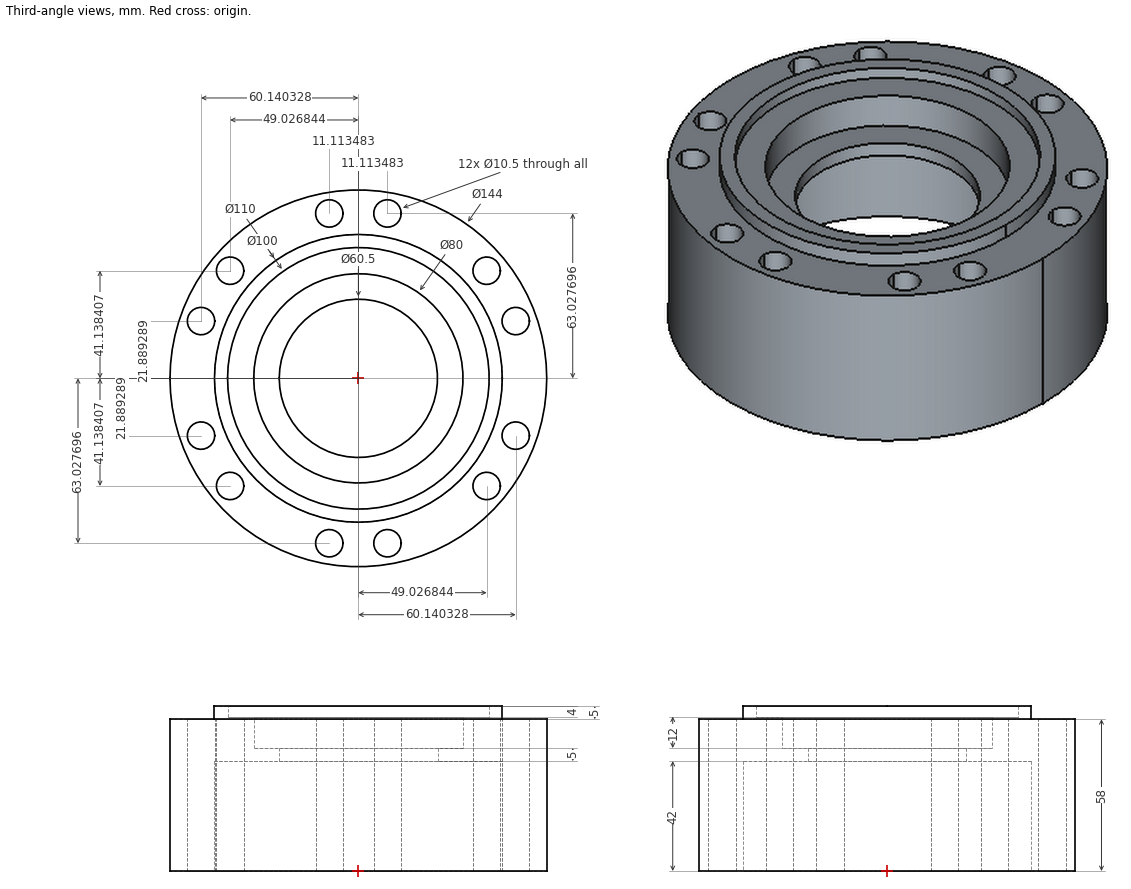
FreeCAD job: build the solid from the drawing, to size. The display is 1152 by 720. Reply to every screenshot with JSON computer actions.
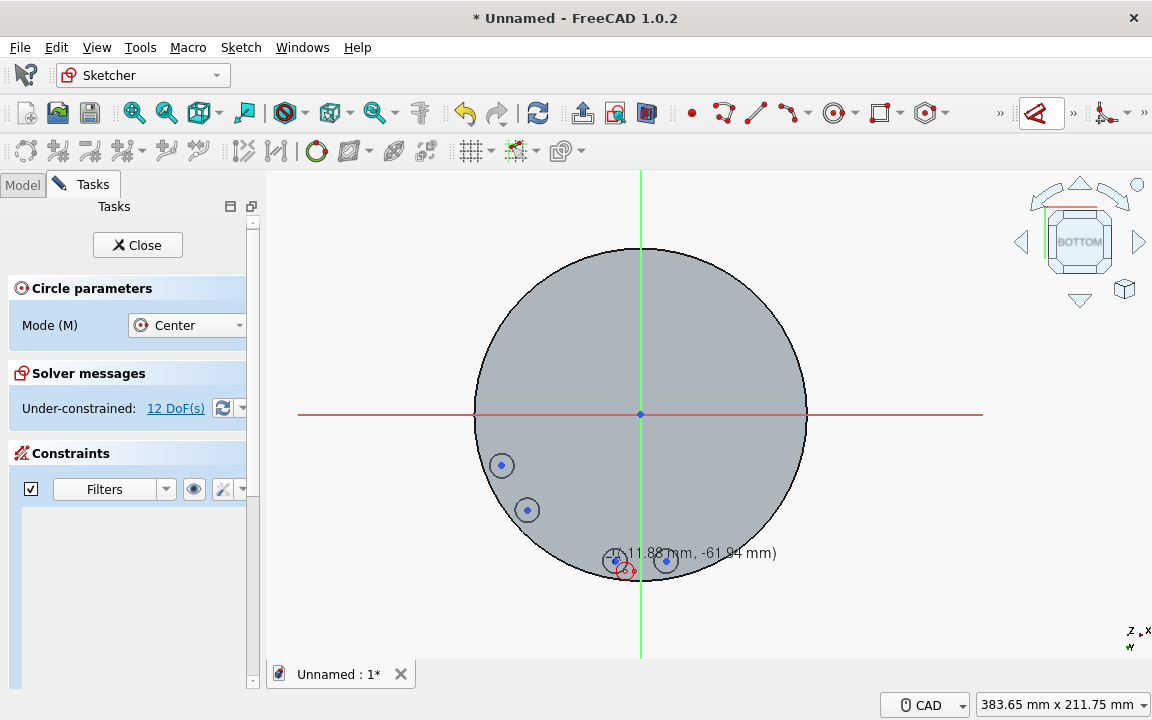
{"action": "scroll", "coordinate": [502, 364], "scroll_direction": "up", "scroll_amount": 4}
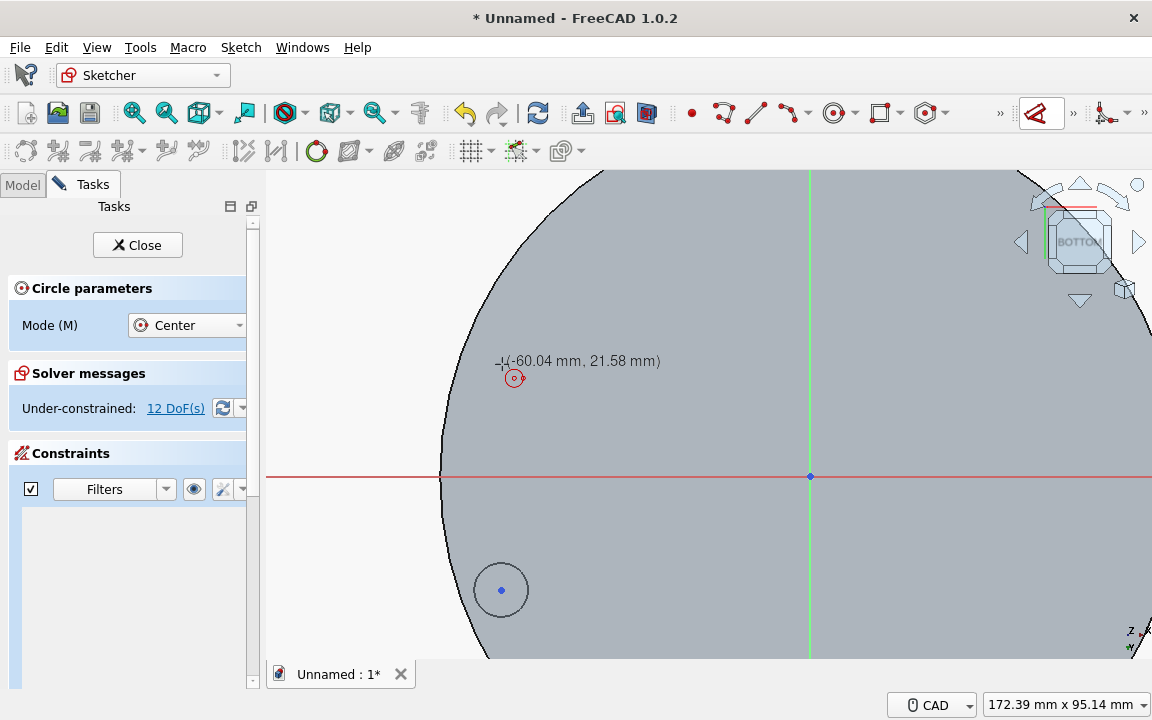
{"action": "left_click", "coordinate": [501, 364]}
{"action": "left_click", "coordinate": [520, 345]}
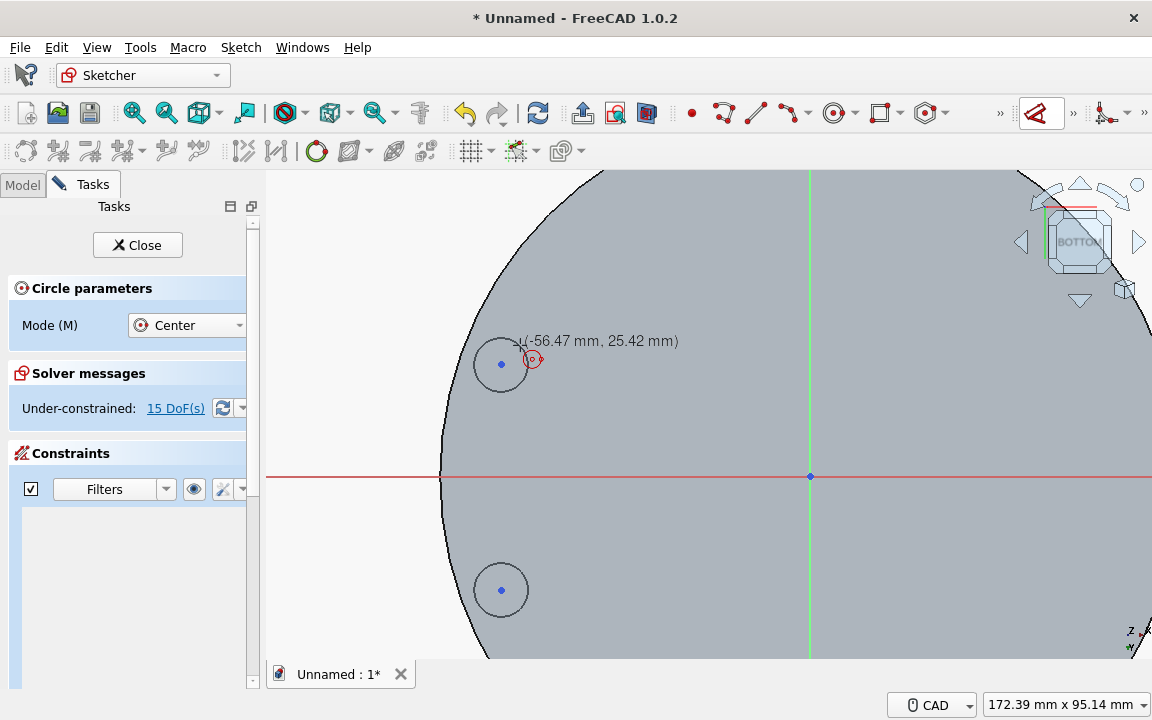
{"action": "left_click", "coordinate": [558, 265]}
{"action": "left_click", "coordinate": [577, 246]}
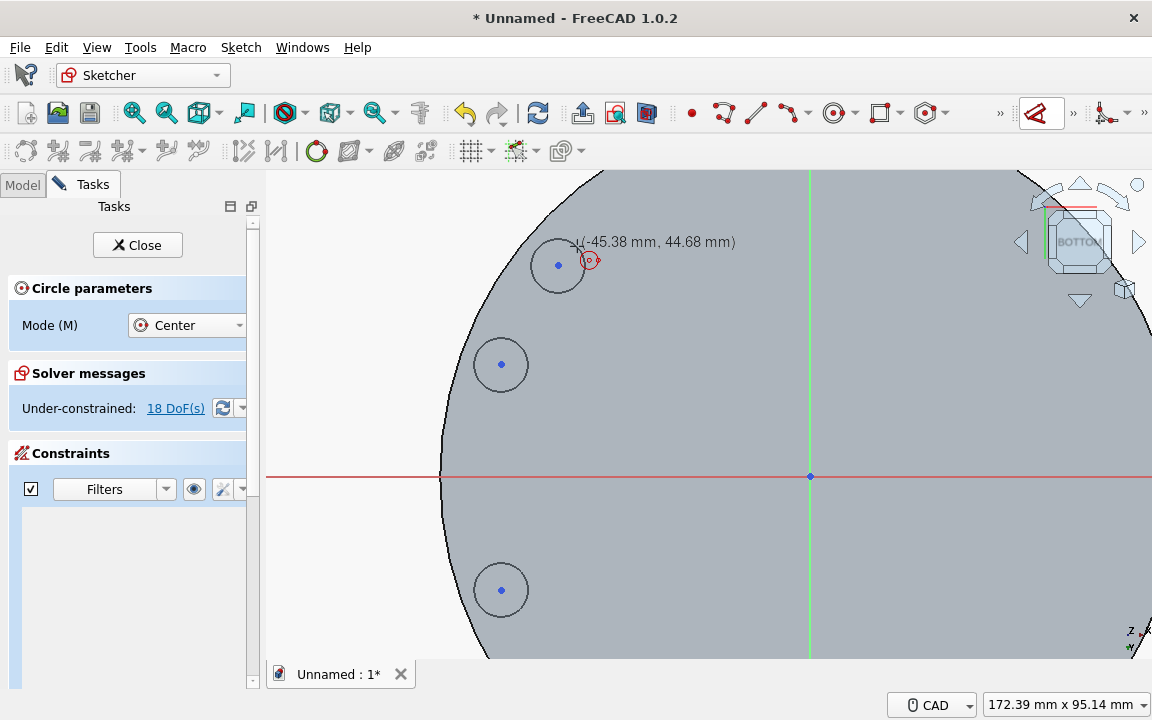
{"action": "scroll", "coordinate": [502, 364], "scroll_direction": "down", "scroll_amount": 4}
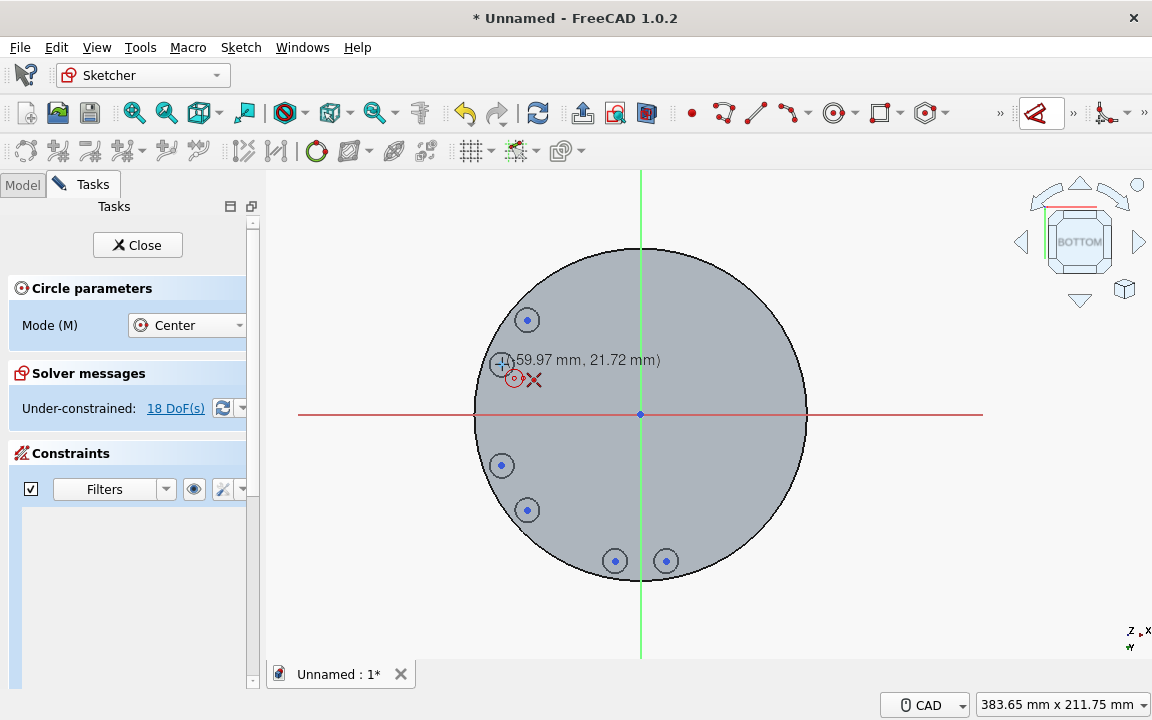
{"action": "scroll", "coordinate": [615, 269], "scroll_direction": "up", "scroll_amount": 4}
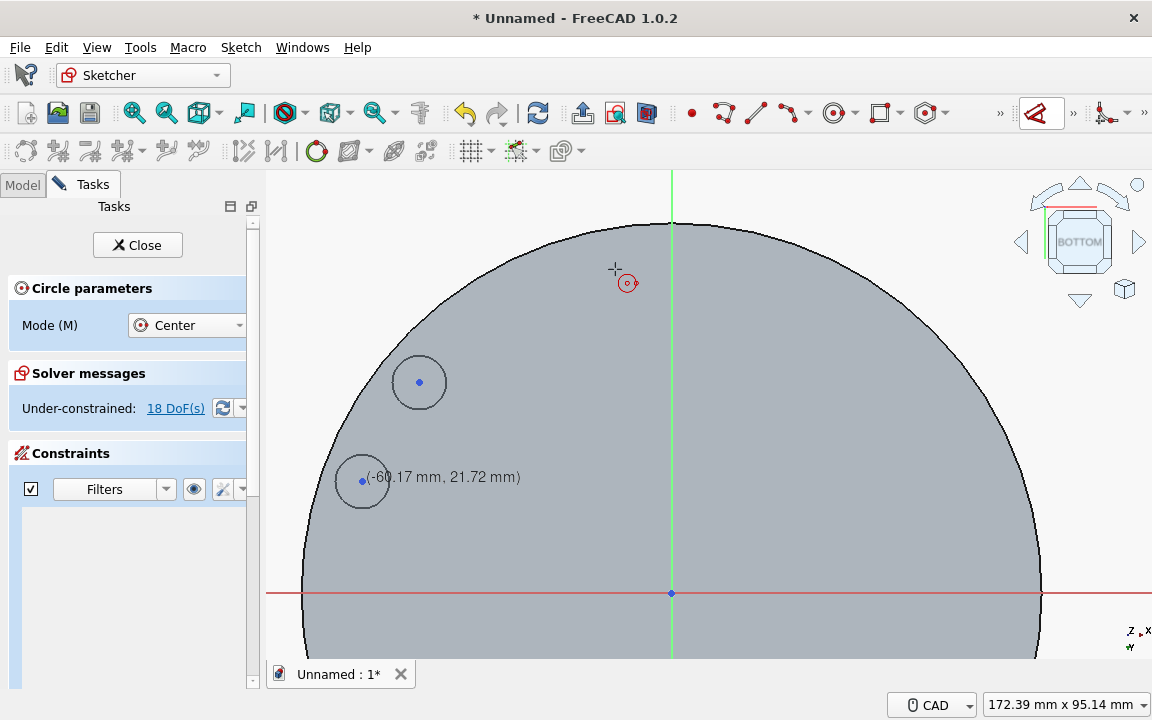
{"action": "left_click", "coordinate": [614, 269]}
{"action": "left_click", "coordinate": [634, 250]}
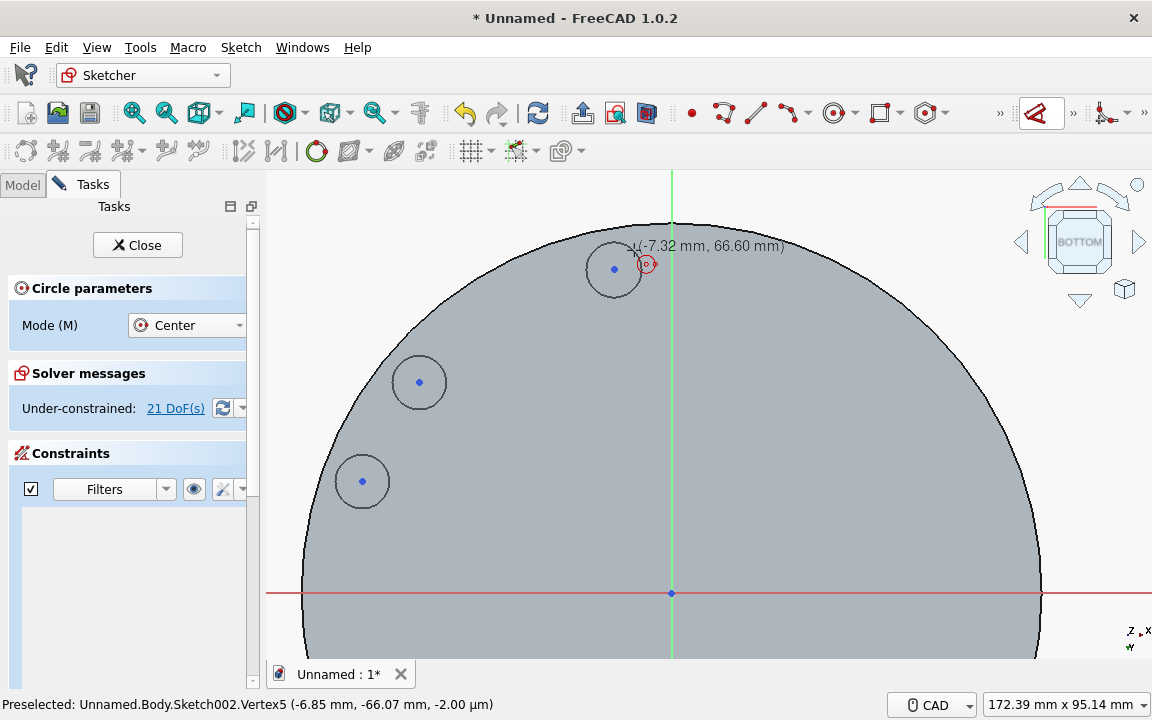
{"action": "left_click", "coordinate": [729, 269]}
{"action": "left_click", "coordinate": [748, 250]}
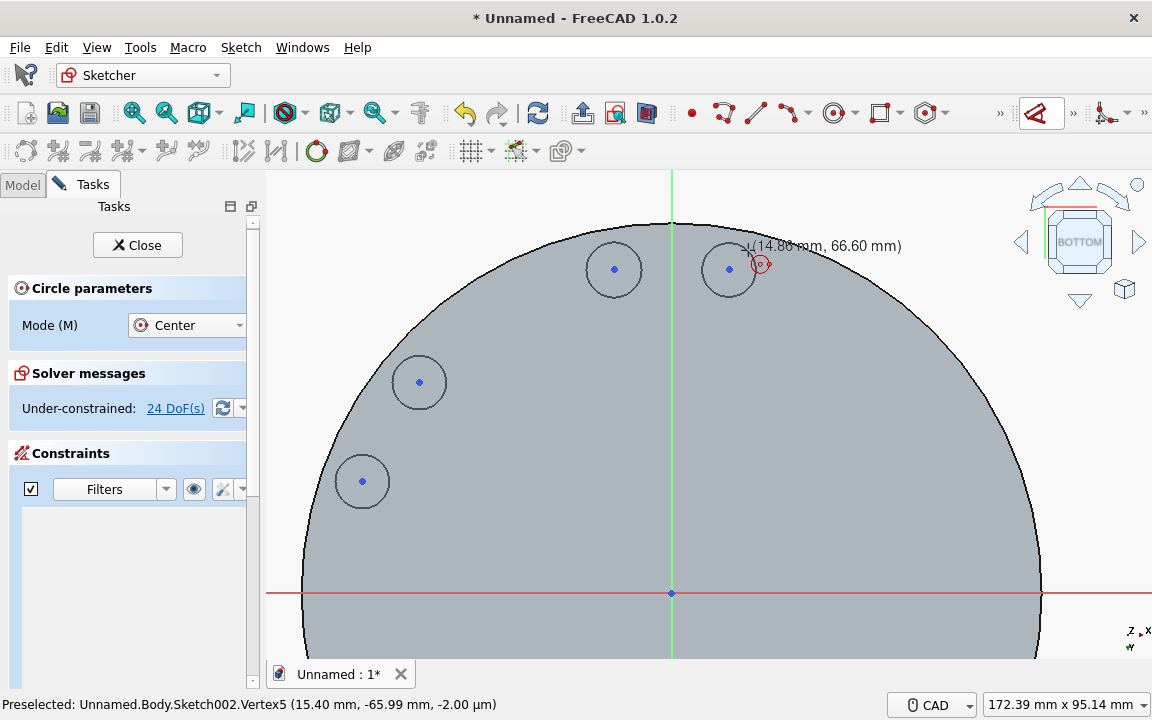
{"action": "left_click", "coordinate": [924, 382]}
{"action": "left_click", "coordinate": [943, 363]}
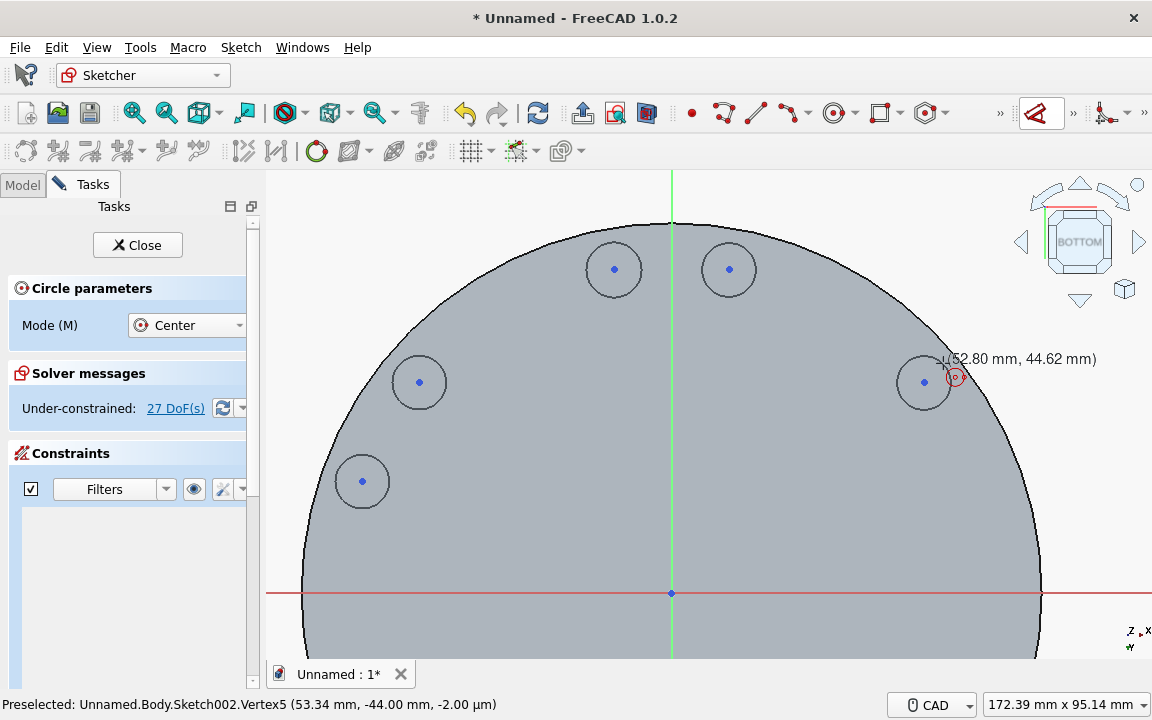
{"action": "left_click", "coordinate": [981, 481]}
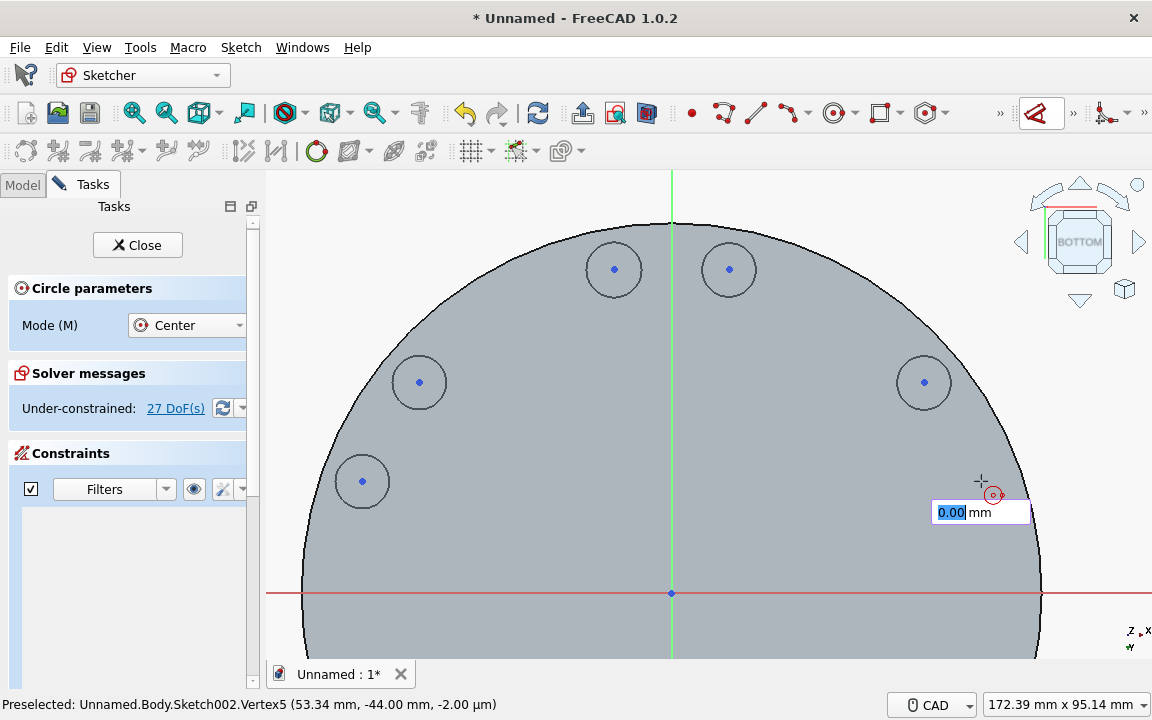
{"action": "scroll", "coordinate": [615, 269], "scroll_direction": "down", "scroll_amount": 4}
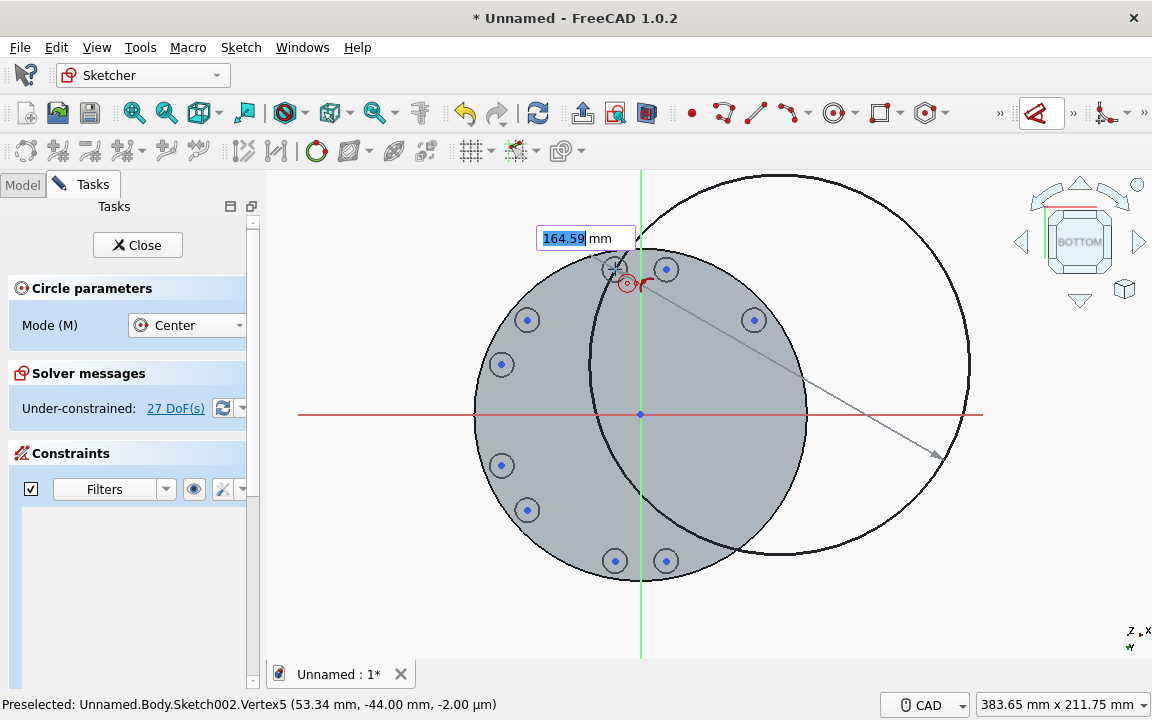
{"action": "scroll", "coordinate": [788, 356], "scroll_direction": "up", "scroll_amount": 2}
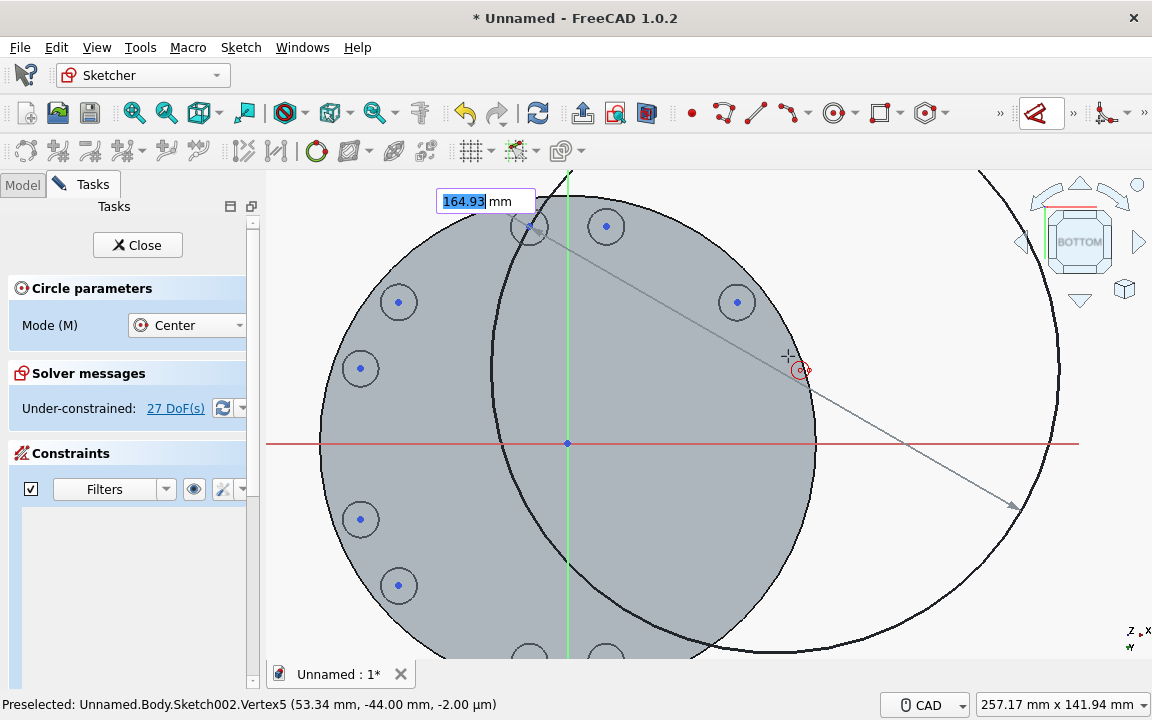
{"action": "left_click", "coordinate": [788, 355]}